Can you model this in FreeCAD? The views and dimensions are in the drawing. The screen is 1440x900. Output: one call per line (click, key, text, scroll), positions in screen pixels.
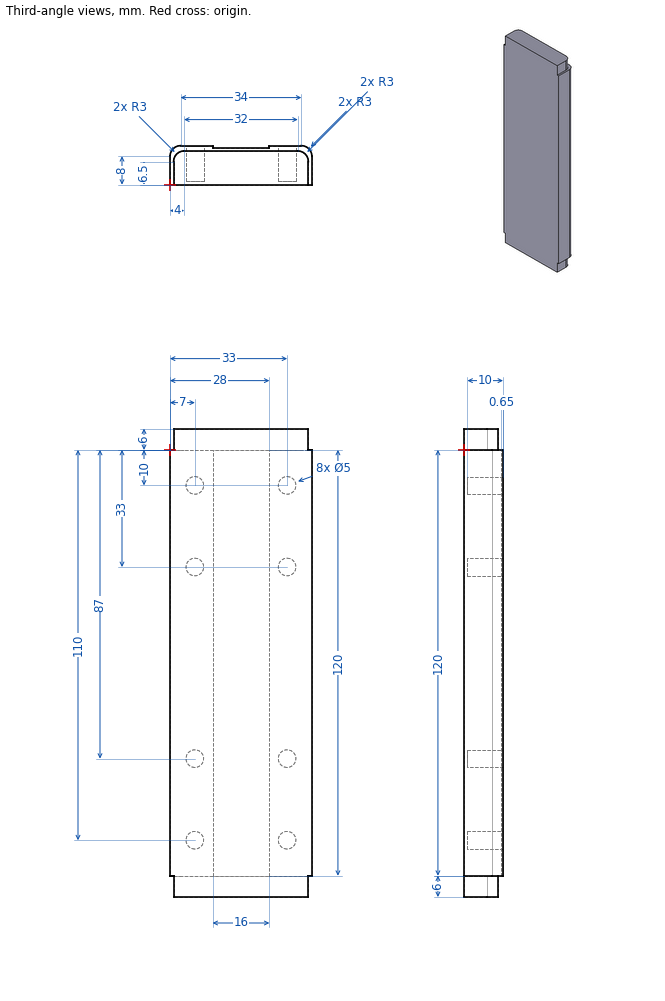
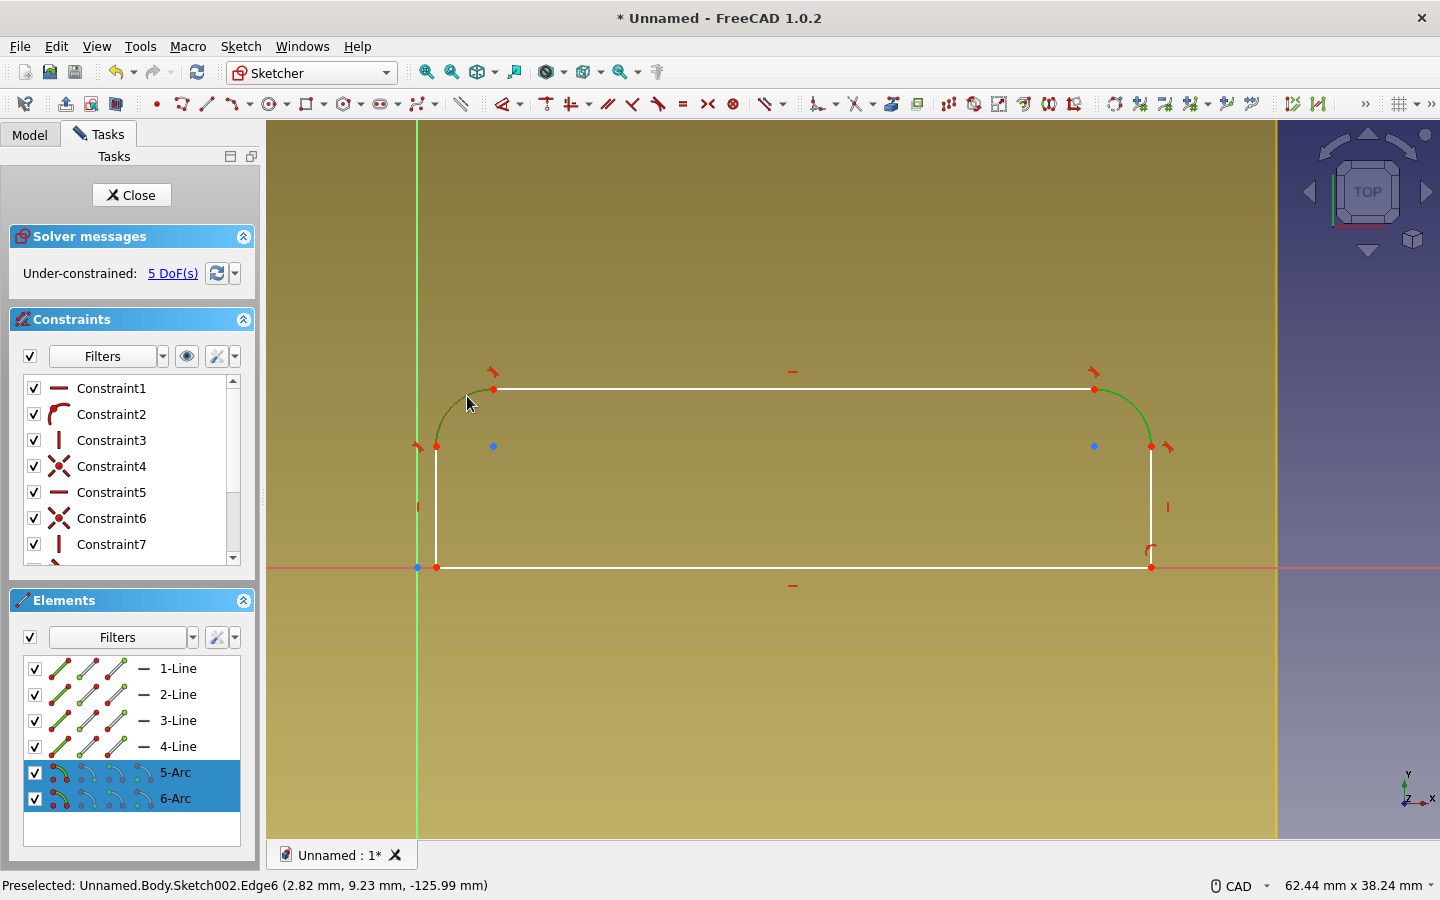
click(683, 104)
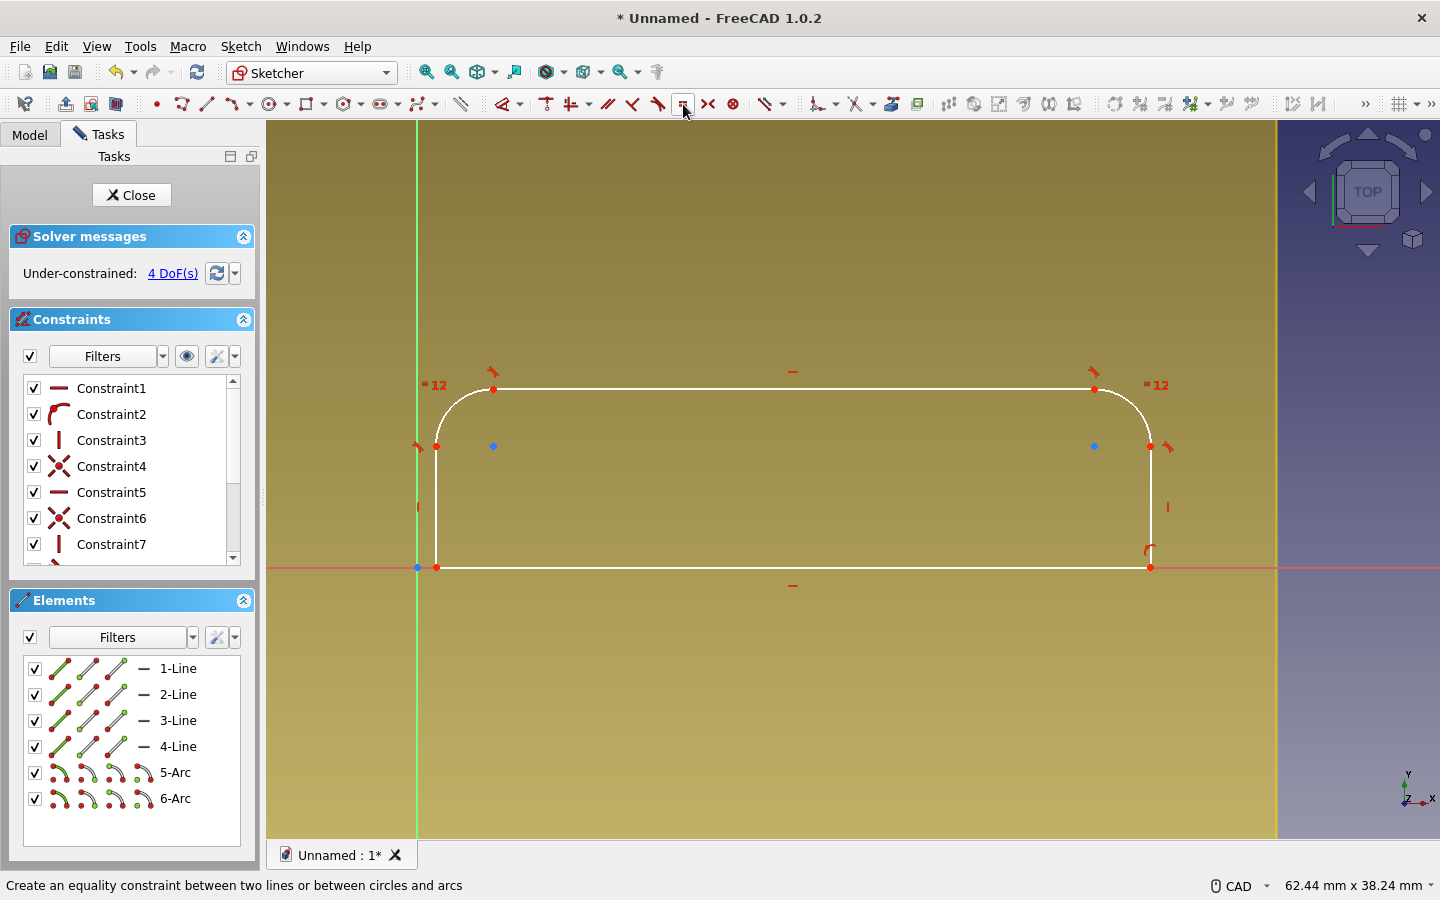
click(502, 104)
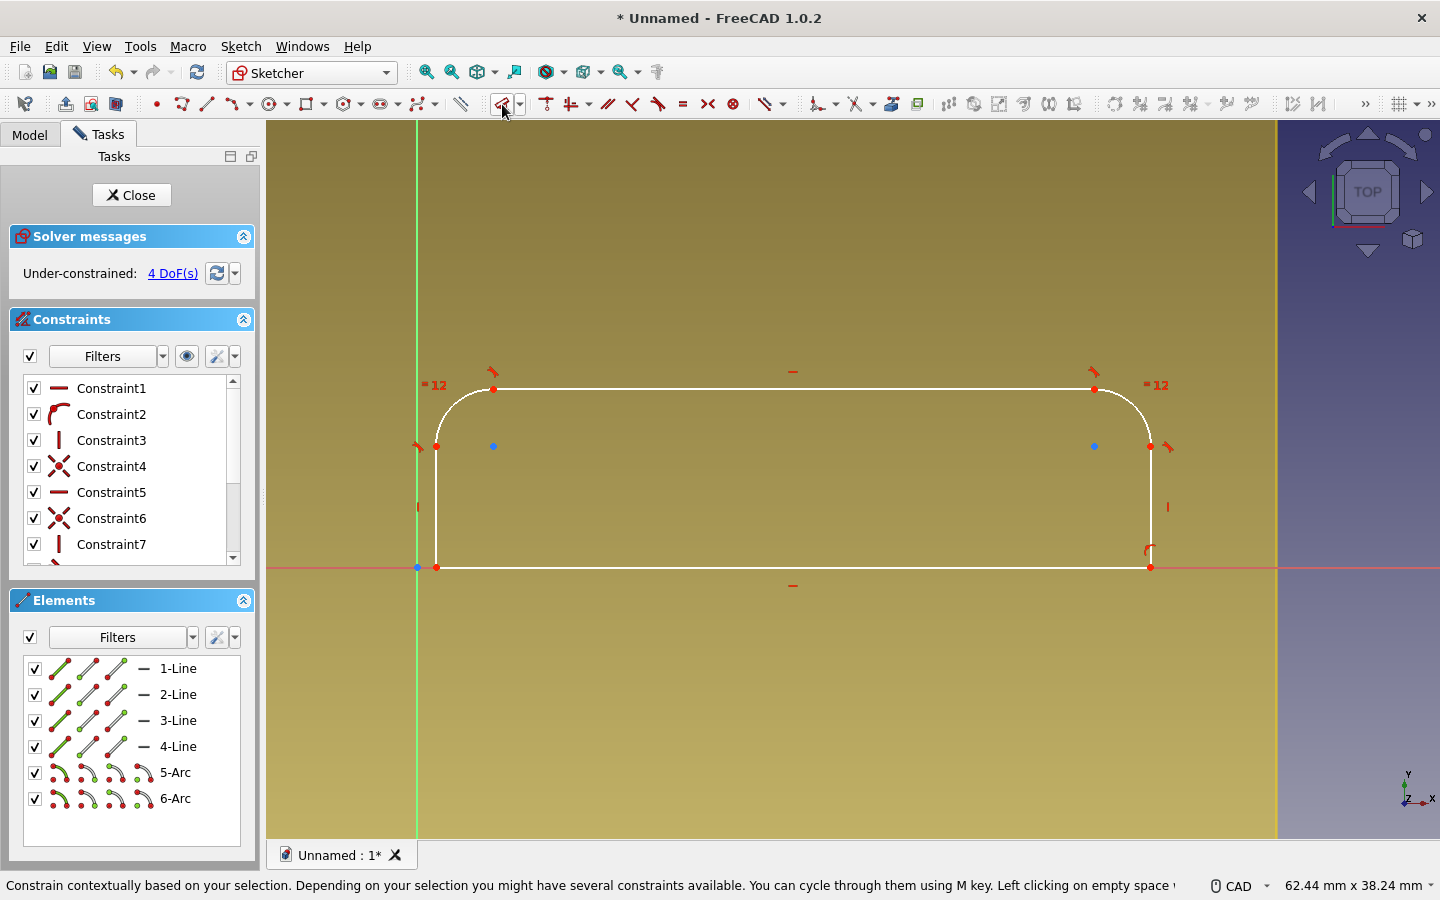
click(1145, 420)
click(1173, 405)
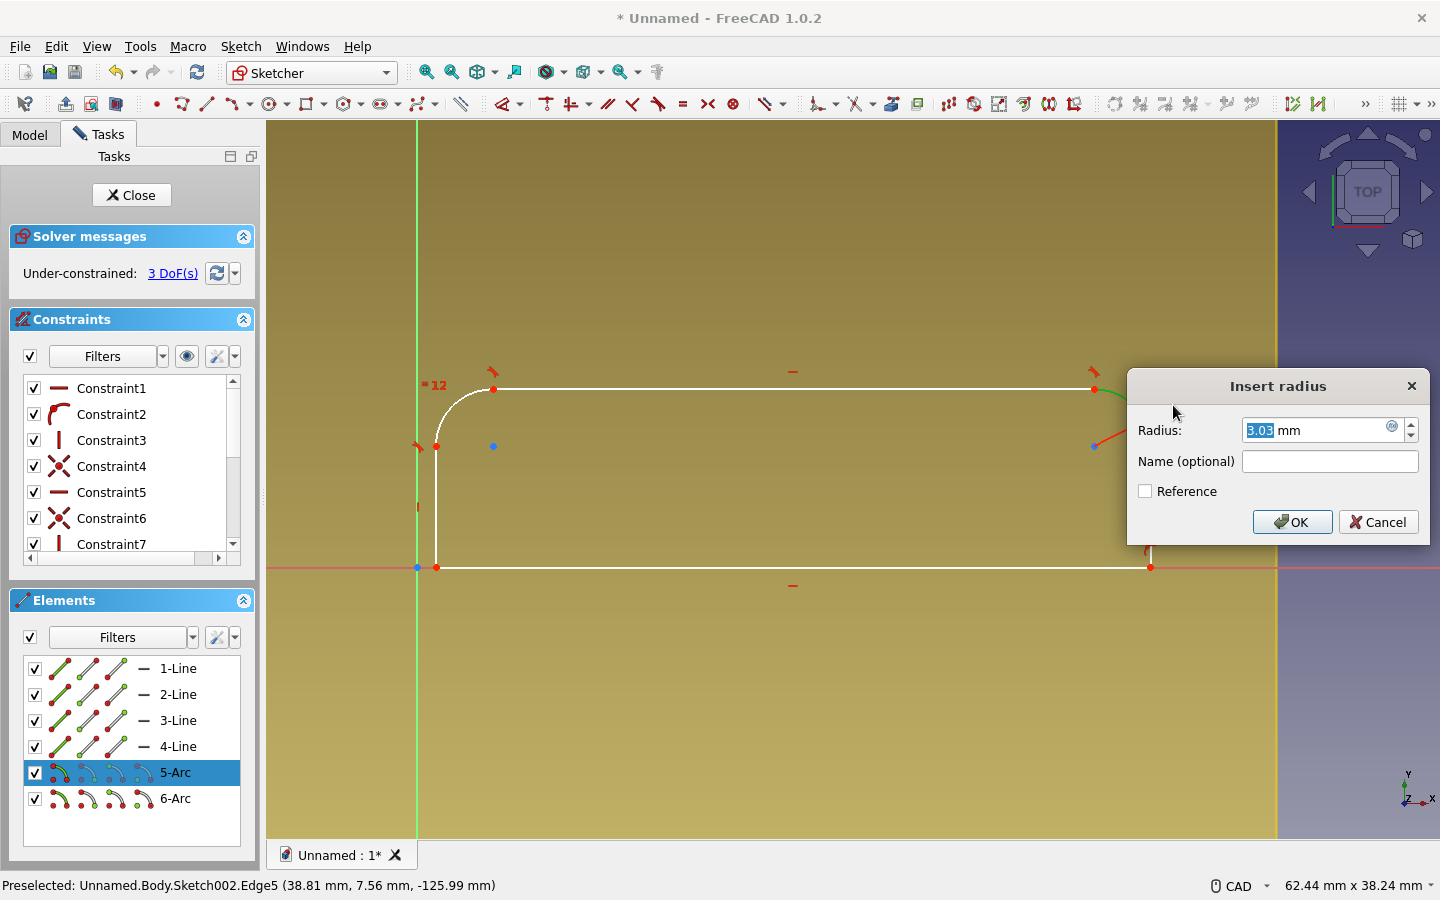
text(3)
key(Return)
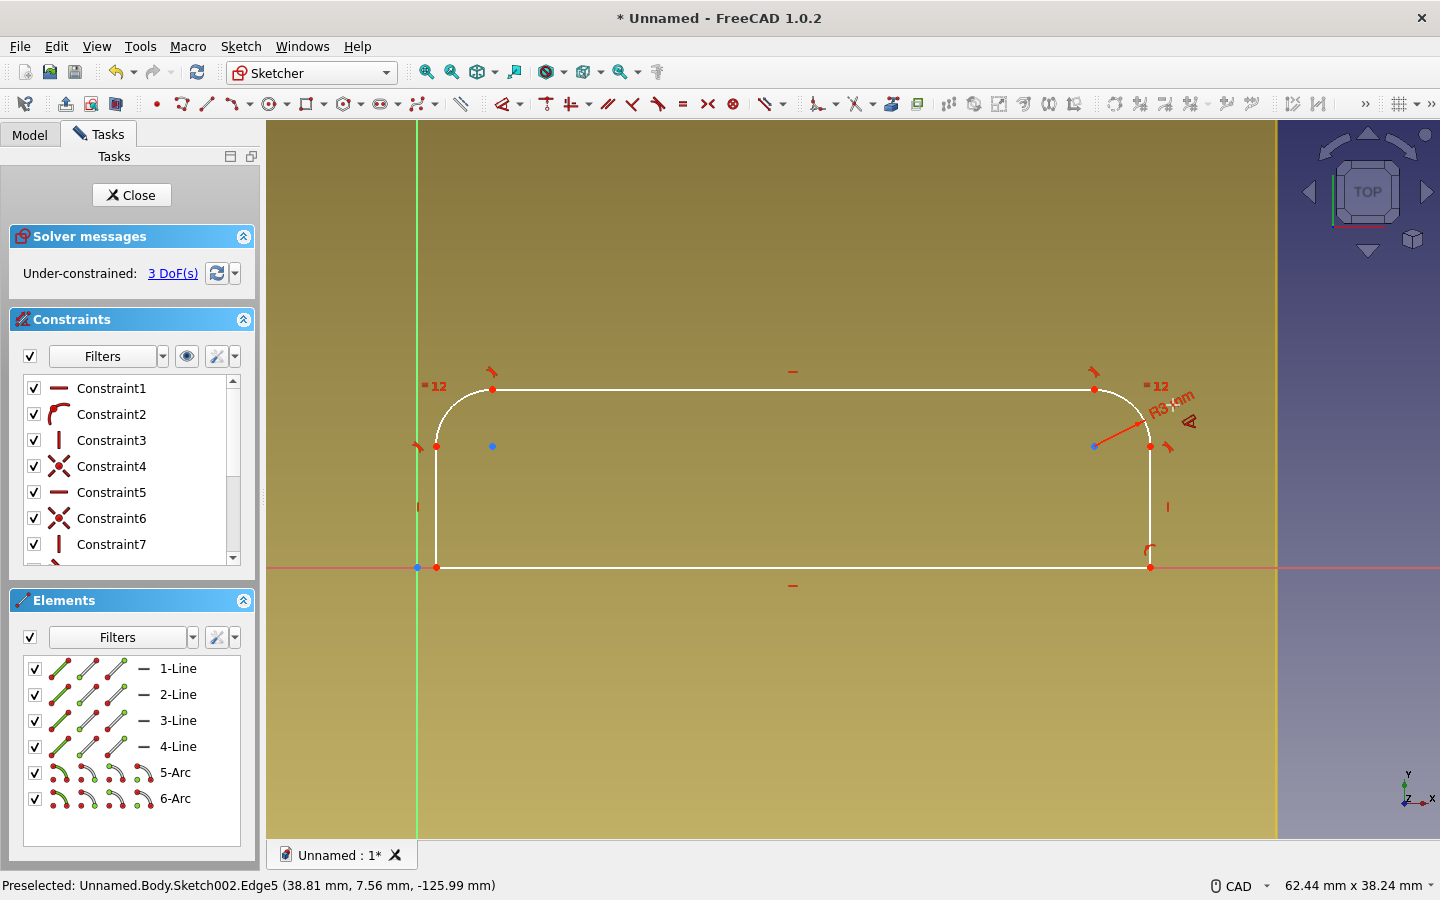
click(673, 390)
click(793, 356)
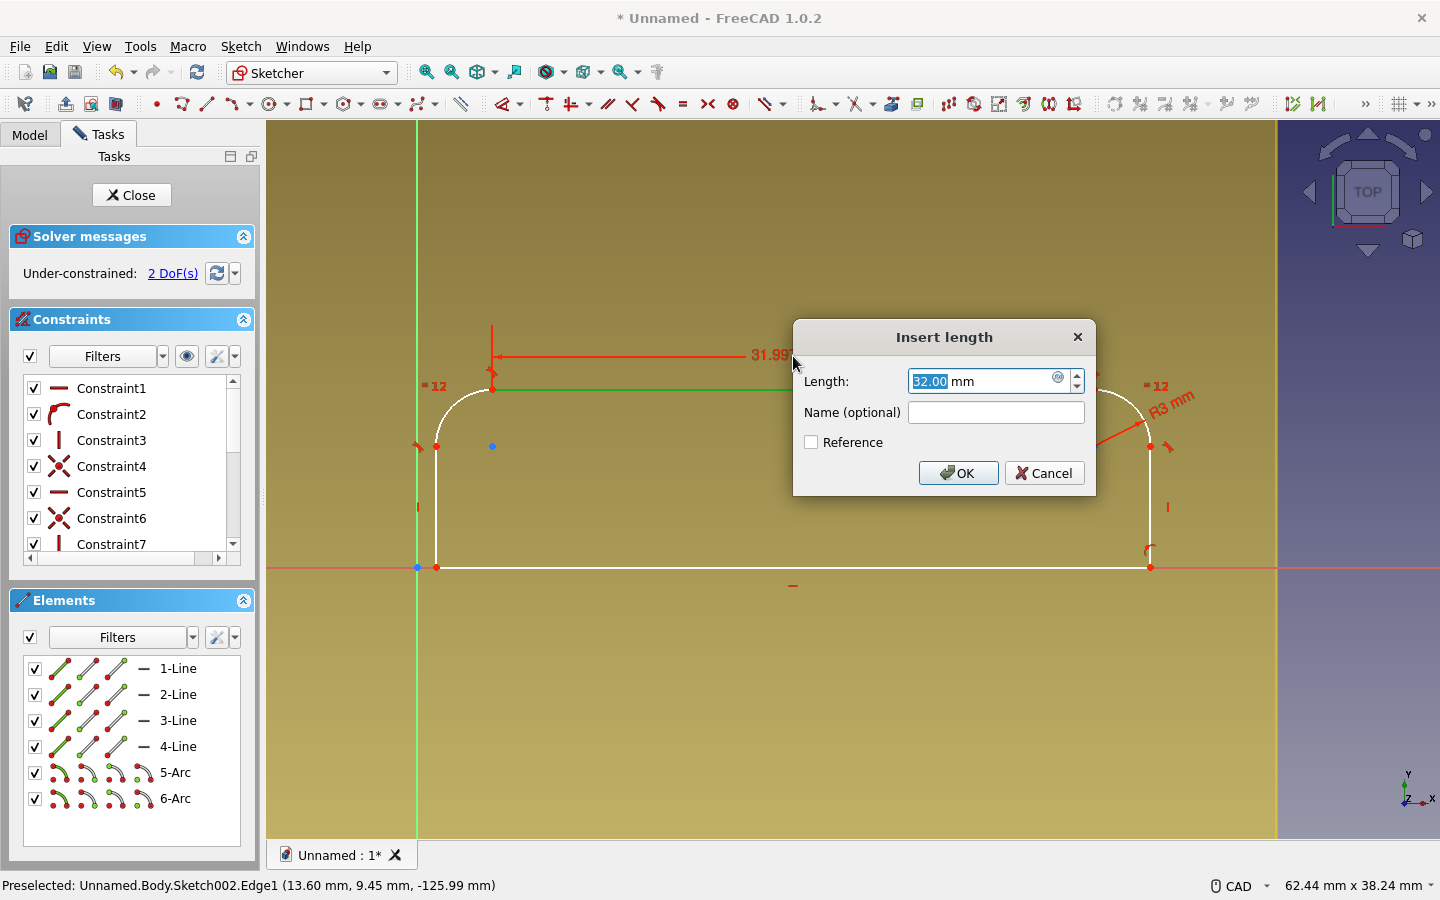
text(32)
key(Return)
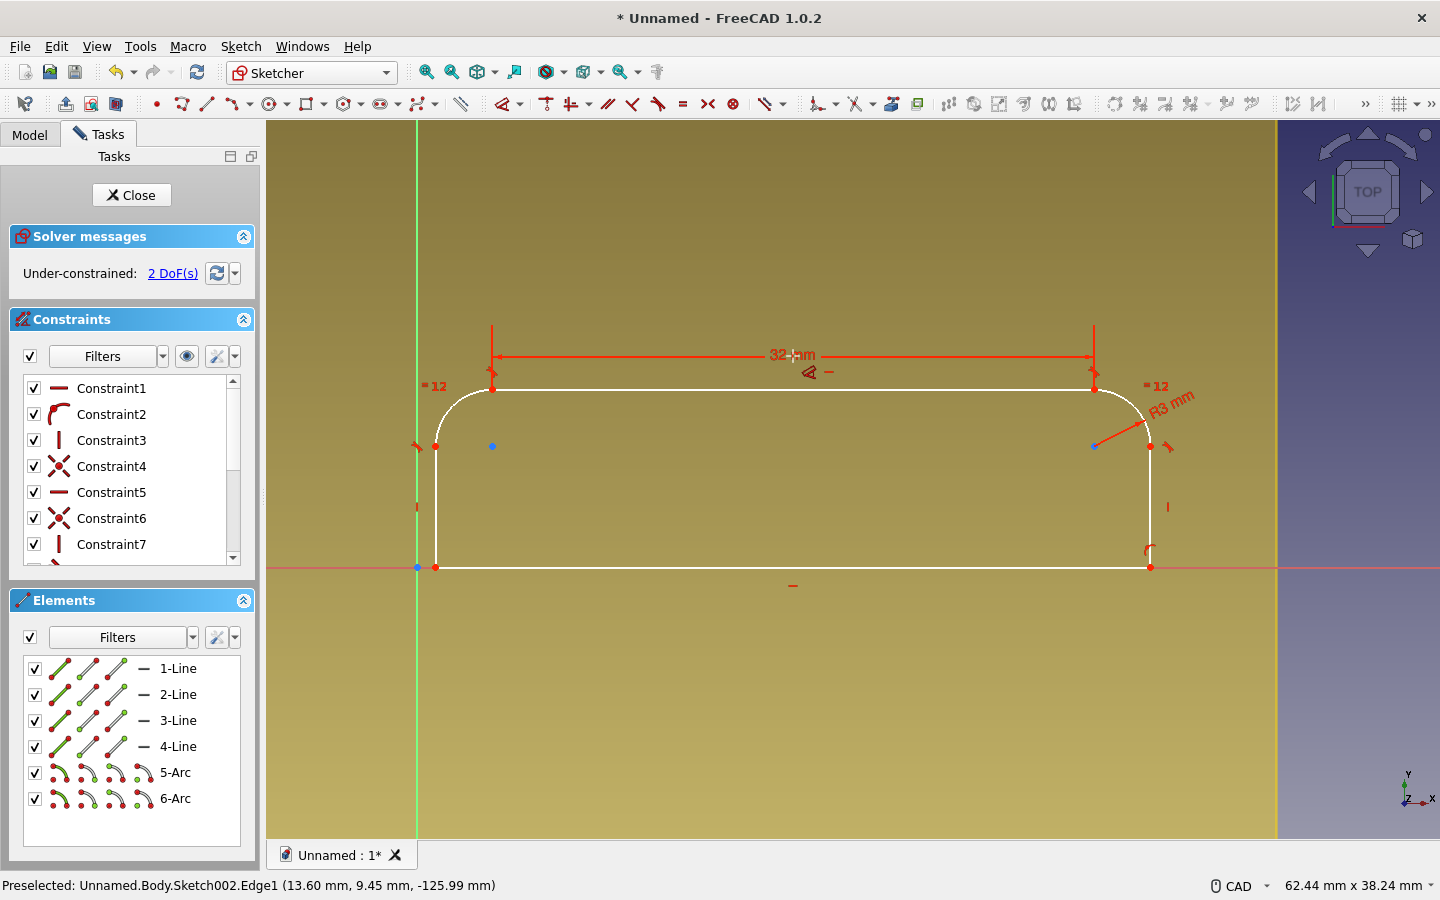
click(492, 390)
click(455, 602)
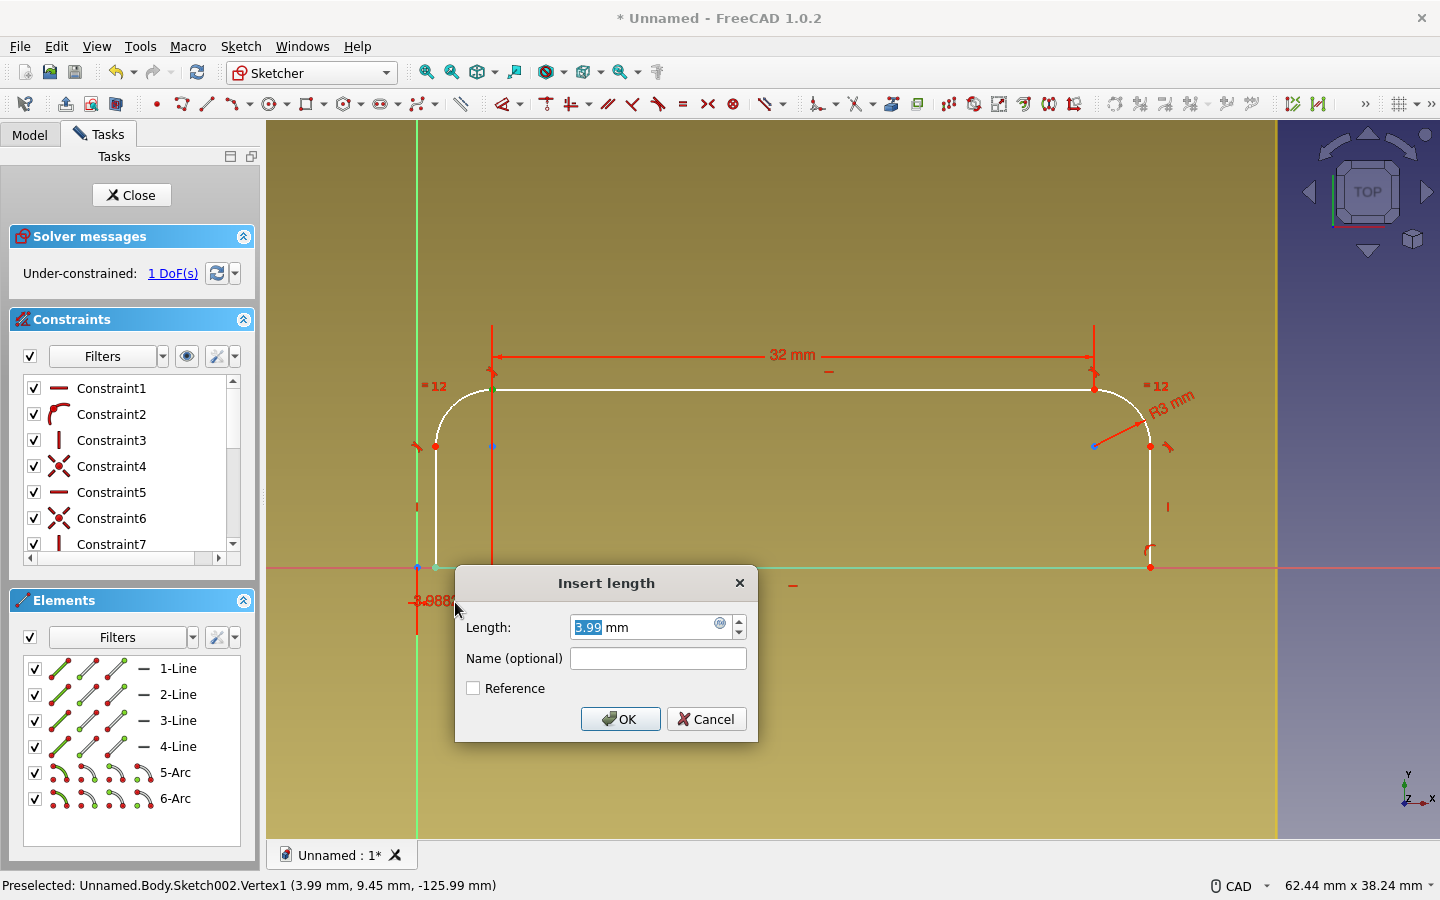
text(4)
key(Return)